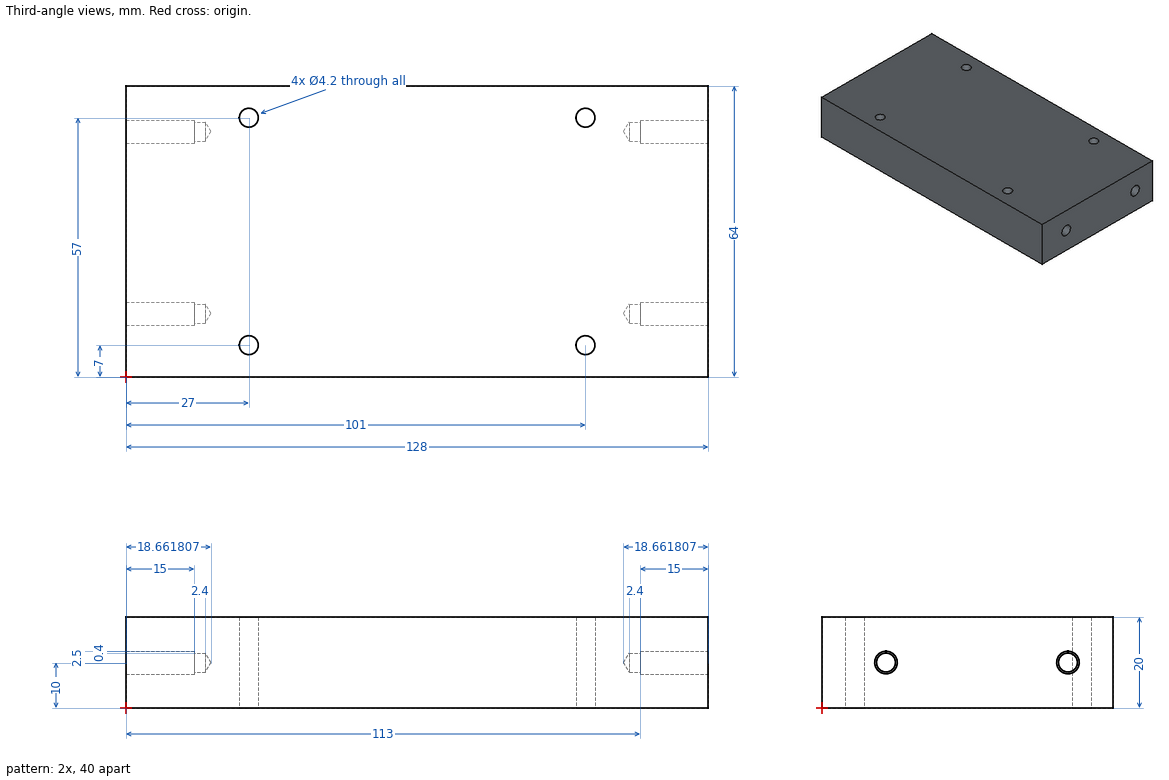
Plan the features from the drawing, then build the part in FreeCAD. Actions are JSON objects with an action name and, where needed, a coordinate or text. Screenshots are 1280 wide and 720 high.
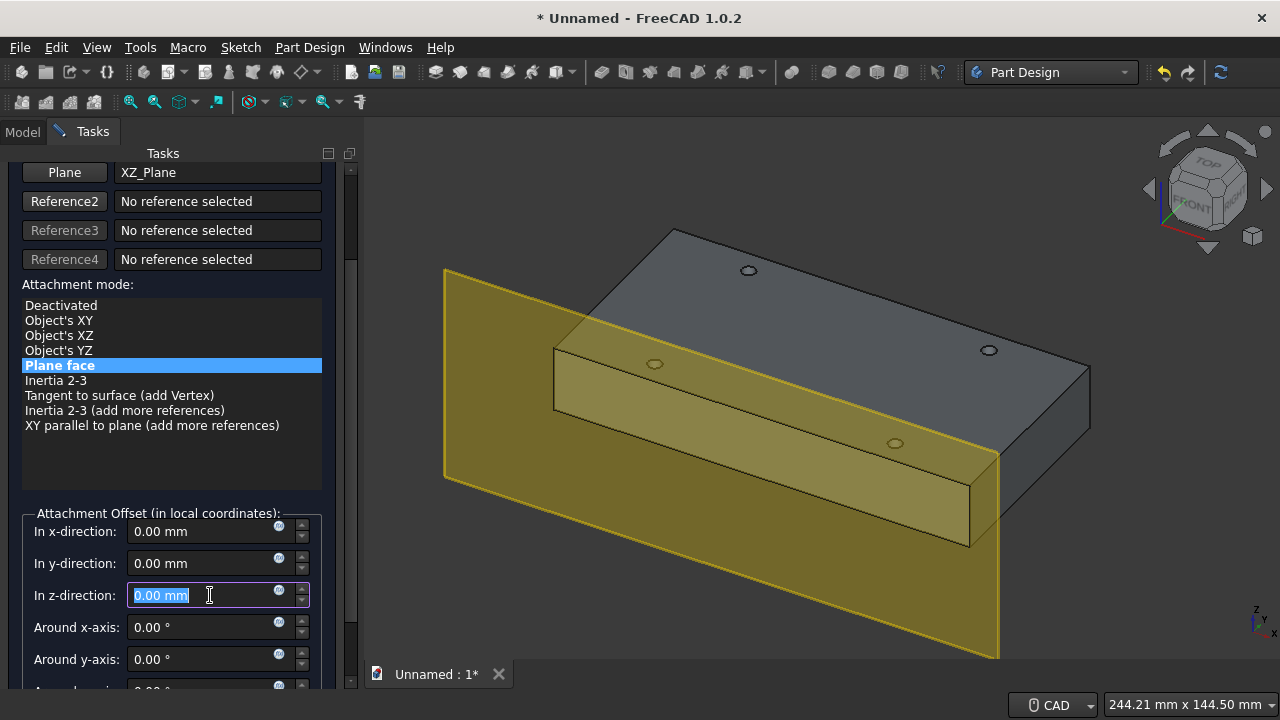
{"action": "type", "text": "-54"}
{"action": "key", "text": "Tab"}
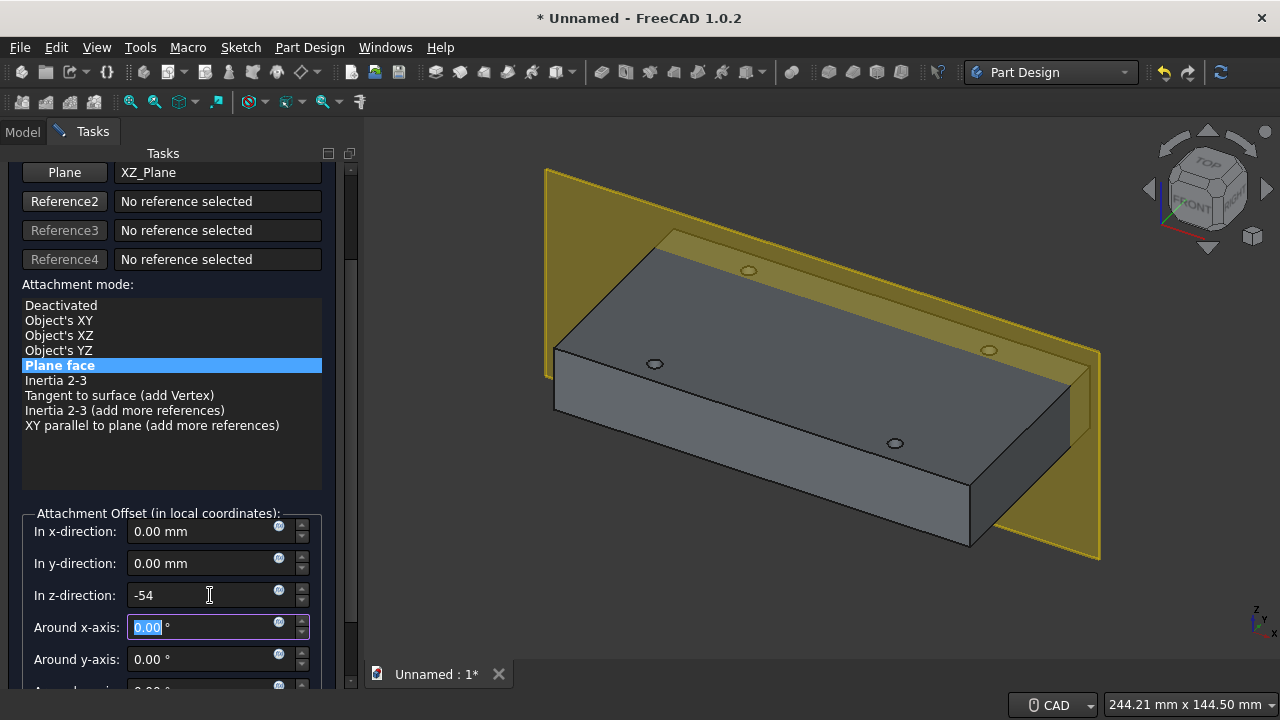
{"action": "scroll", "coordinate": [351, 426], "scroll_direction": "up", "scroll_amount": 3}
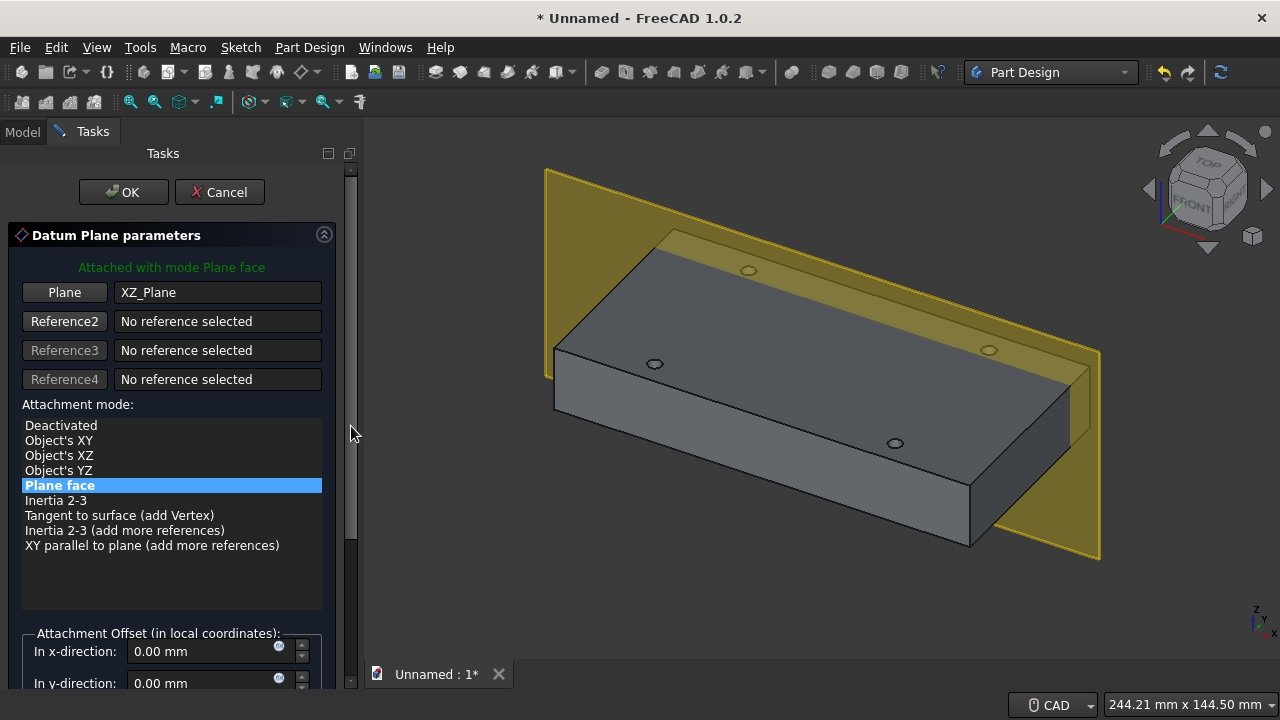
{"action": "left_click", "coordinate": [124, 192]}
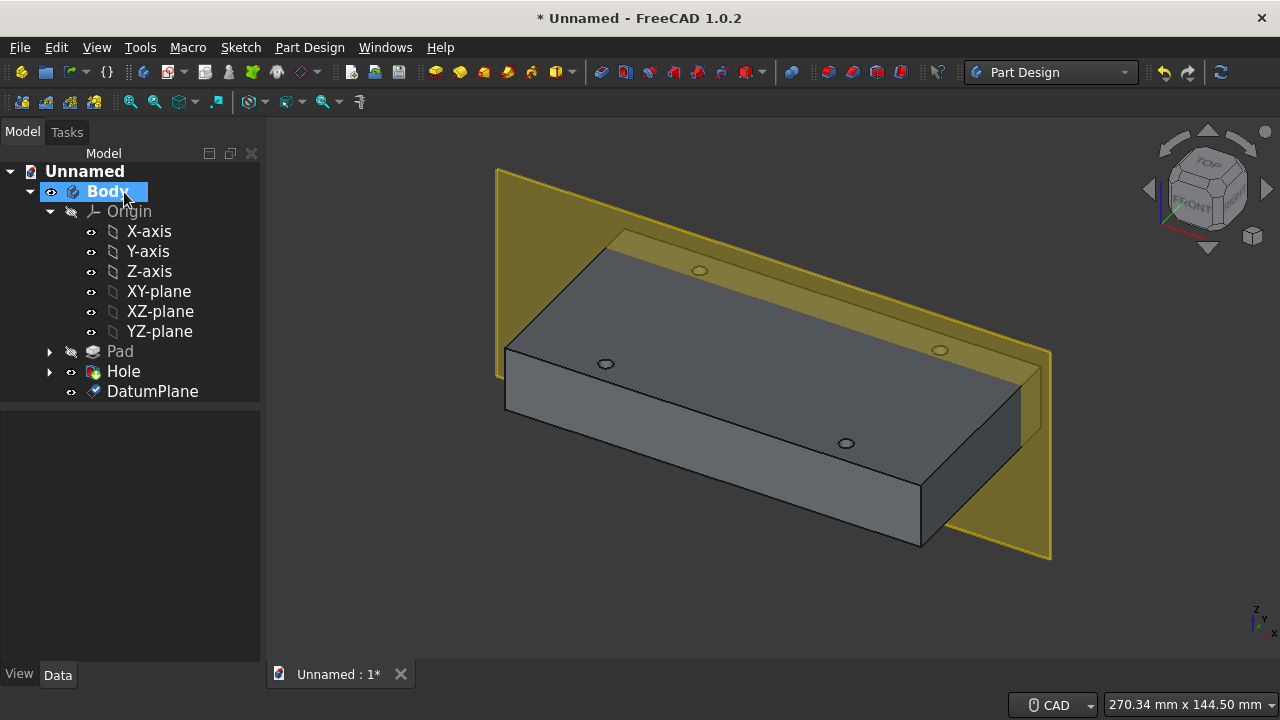
{"action": "left_click", "coordinate": [116, 392]}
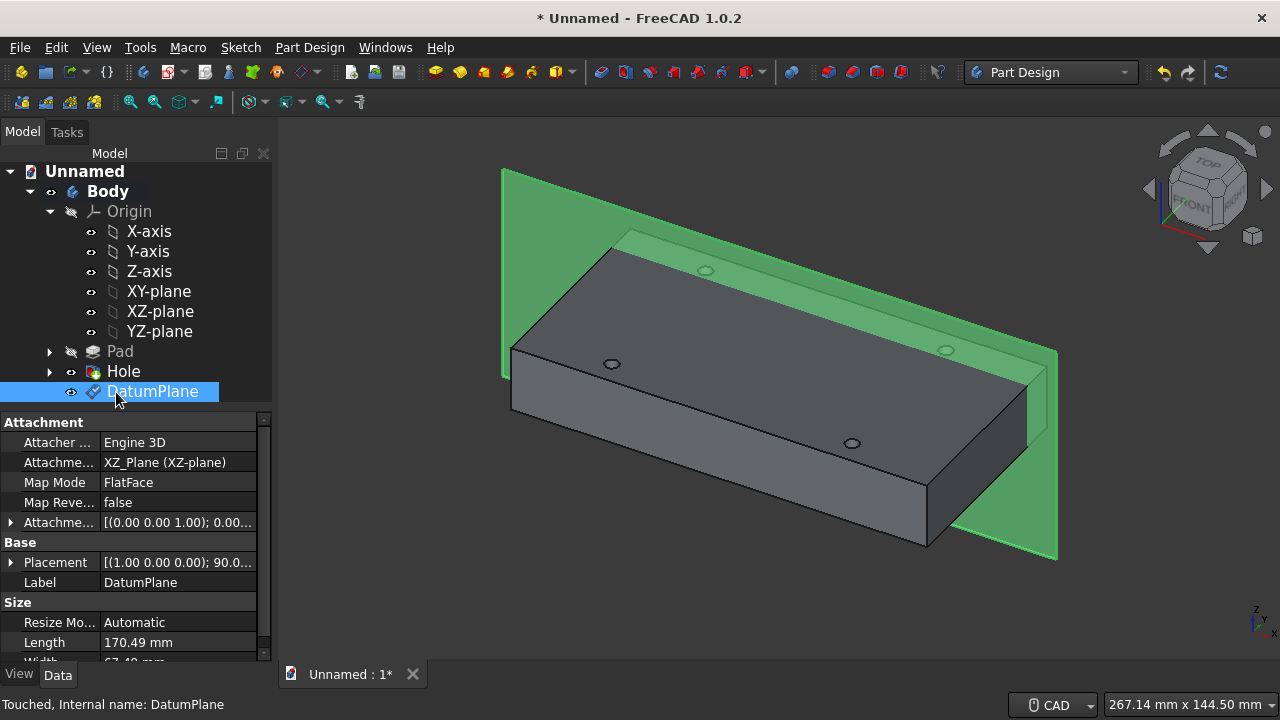
{"action": "left_click", "coordinate": [168, 72]}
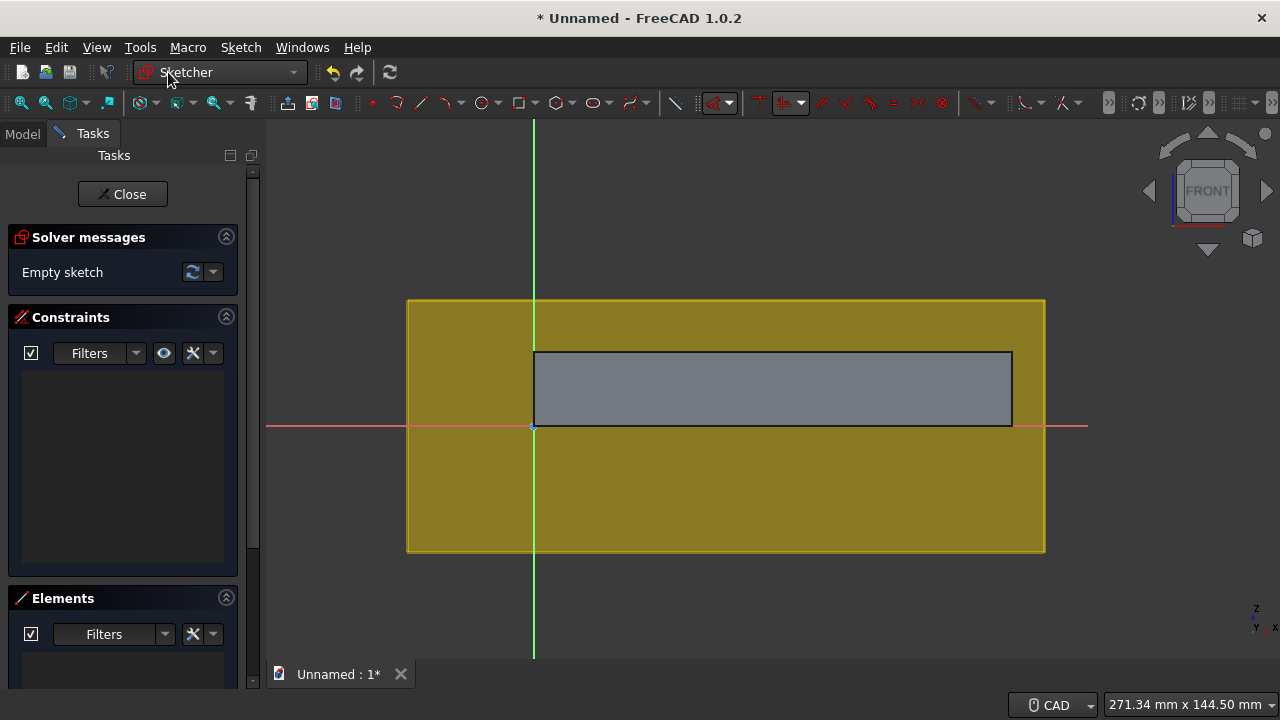
{"action": "left_click", "coordinate": [336, 104]}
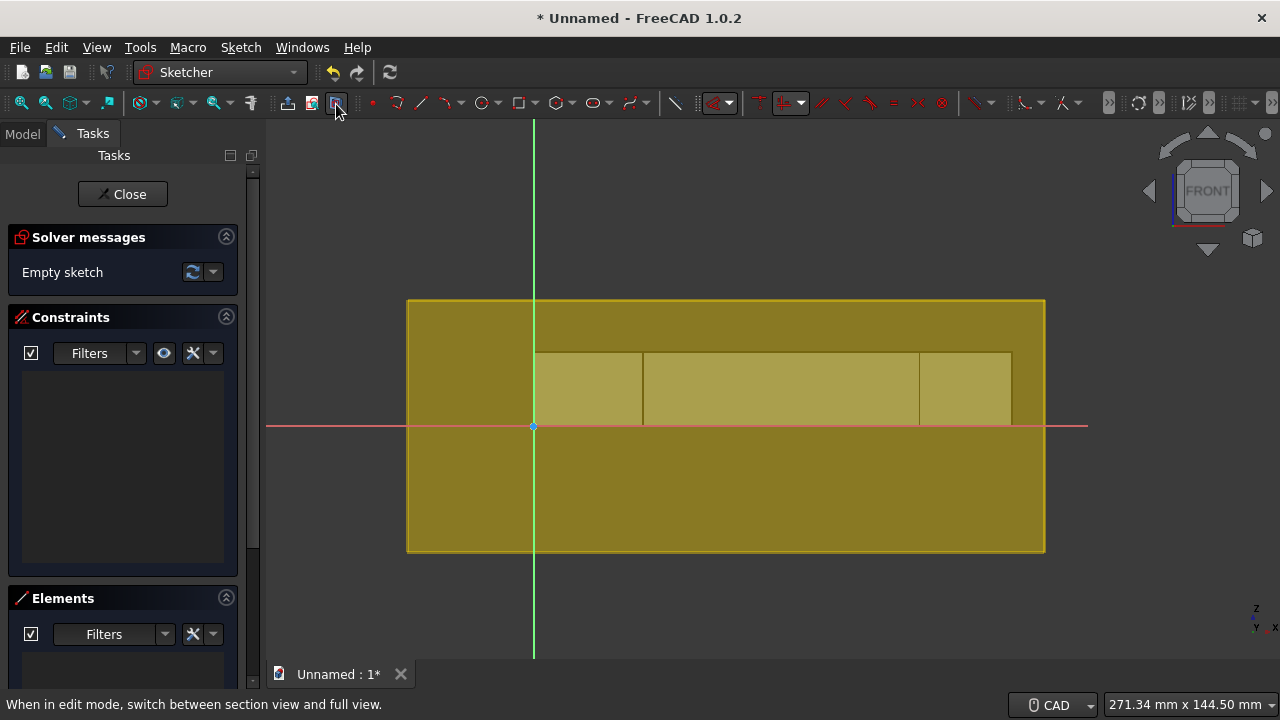
{"action": "scroll", "coordinate": [559, 406], "scroll_direction": "up", "scroll_amount": 9}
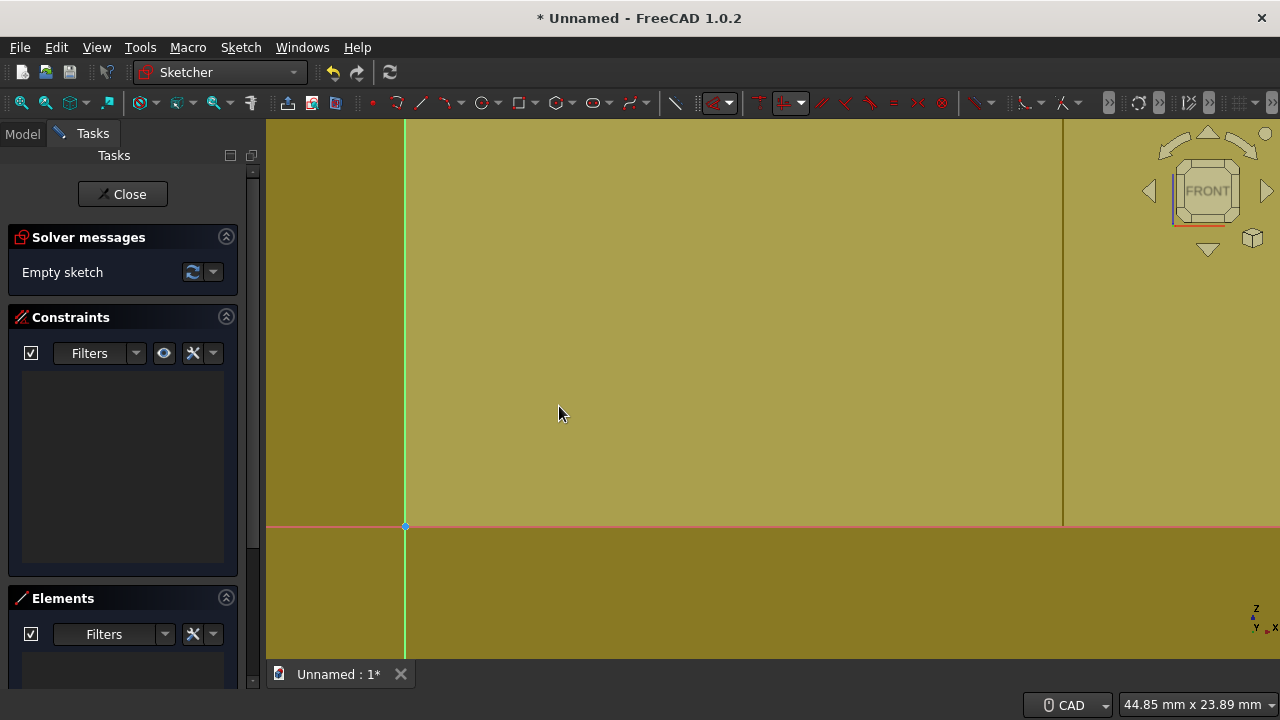
{"action": "left_click", "coordinate": [398, 104]}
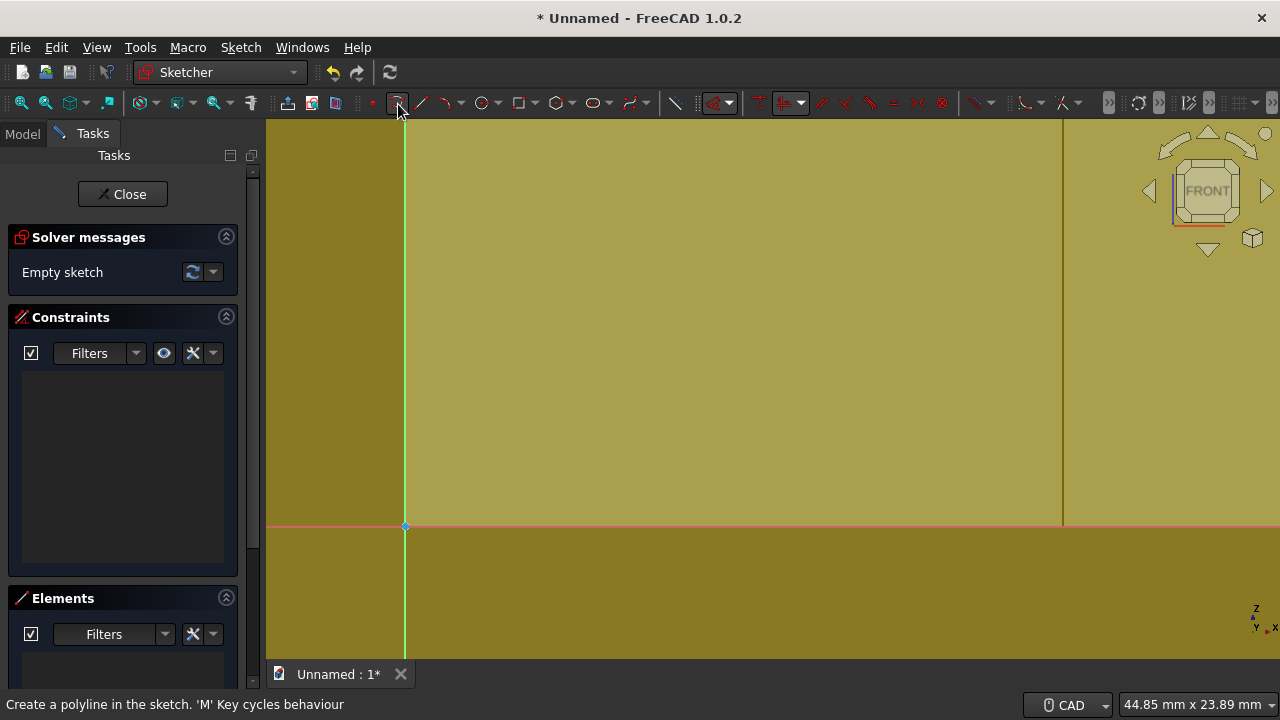
{"action": "left_click", "coordinate": [405, 300]}
{"action": "left_click", "coordinate": [414, 244]}
{"action": "left_click", "coordinate": [744, 244]}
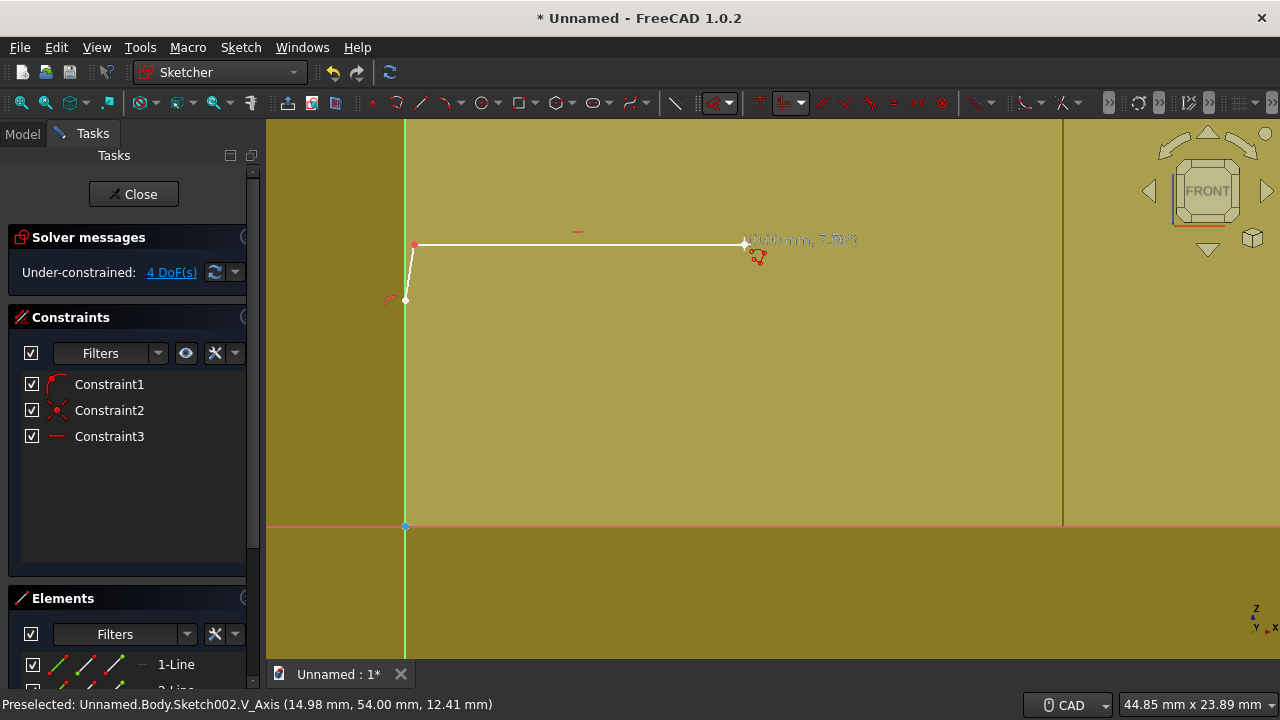
{"action": "scroll", "coordinate": [744, 253], "scroll_direction": "up", "scroll_amount": 3}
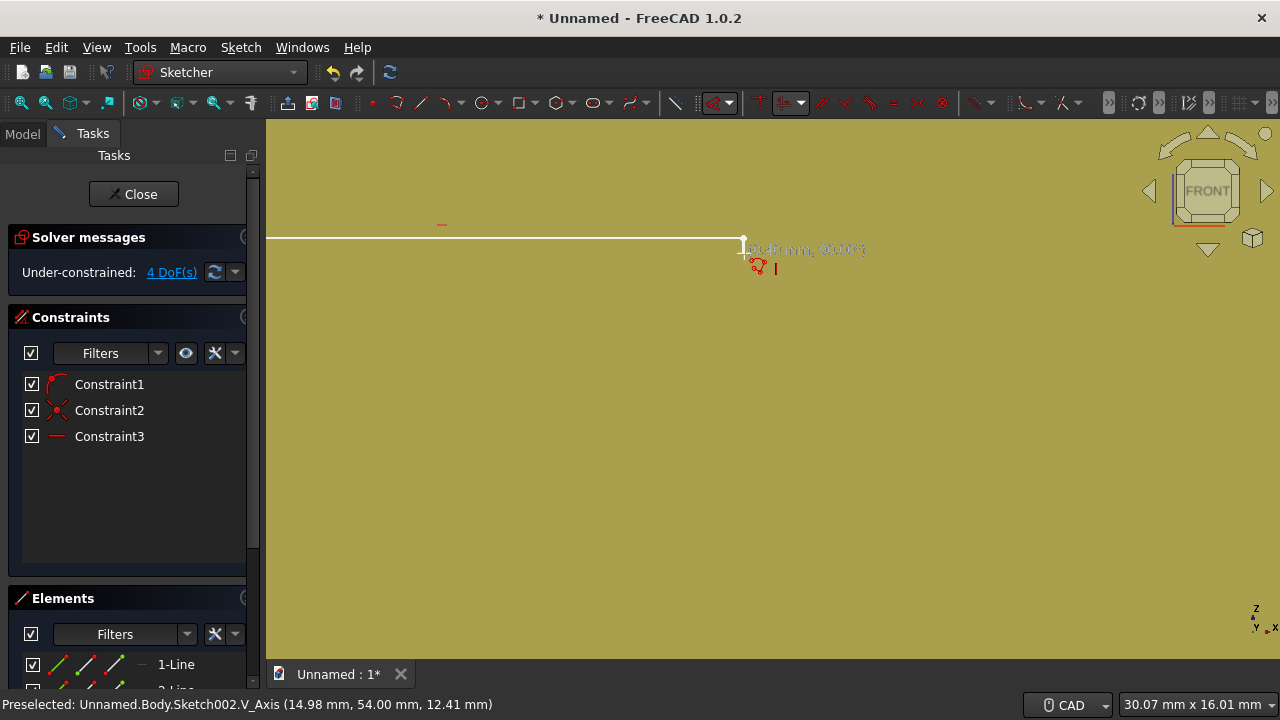
{"action": "left_click", "coordinate": [744, 253]}
{"action": "left_click", "coordinate": [843, 253]}
{"action": "left_click", "coordinate": [895, 339]}